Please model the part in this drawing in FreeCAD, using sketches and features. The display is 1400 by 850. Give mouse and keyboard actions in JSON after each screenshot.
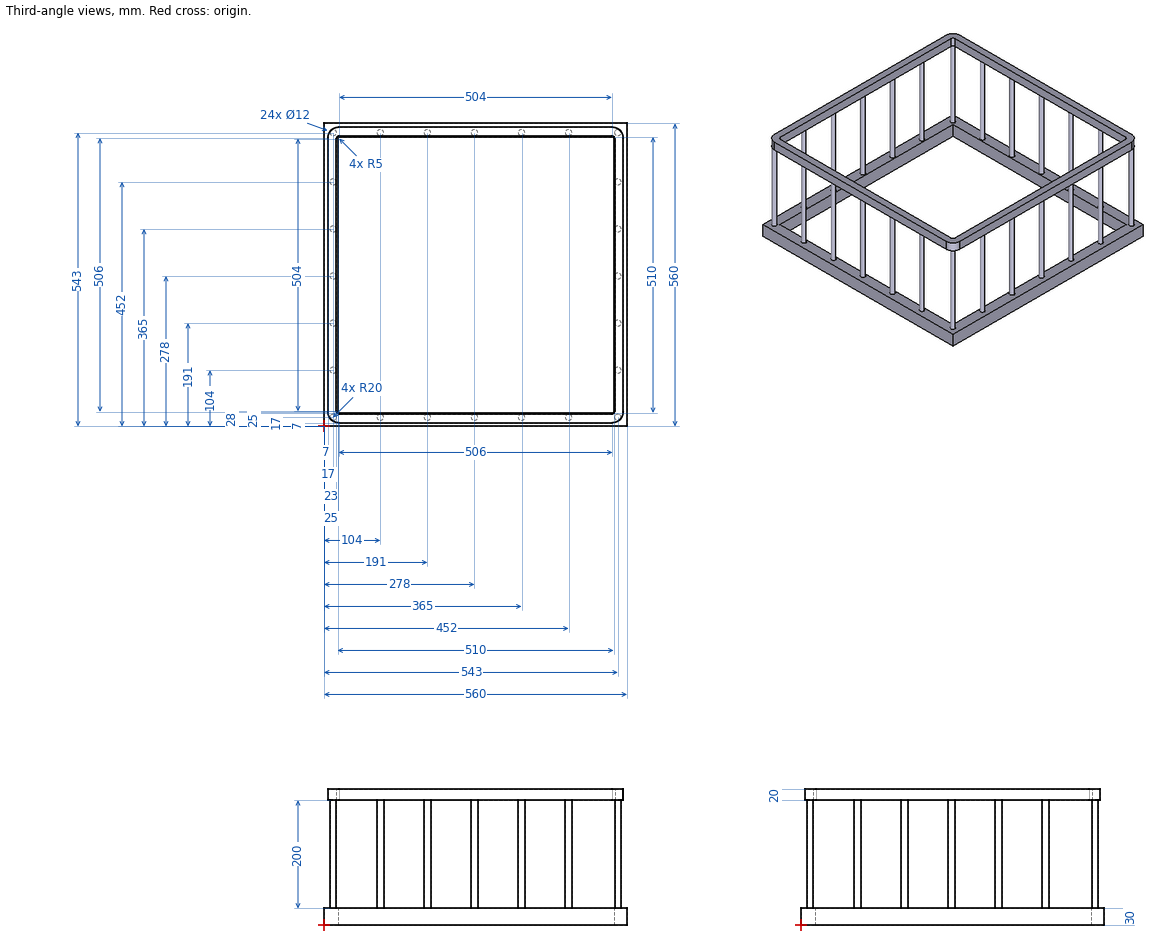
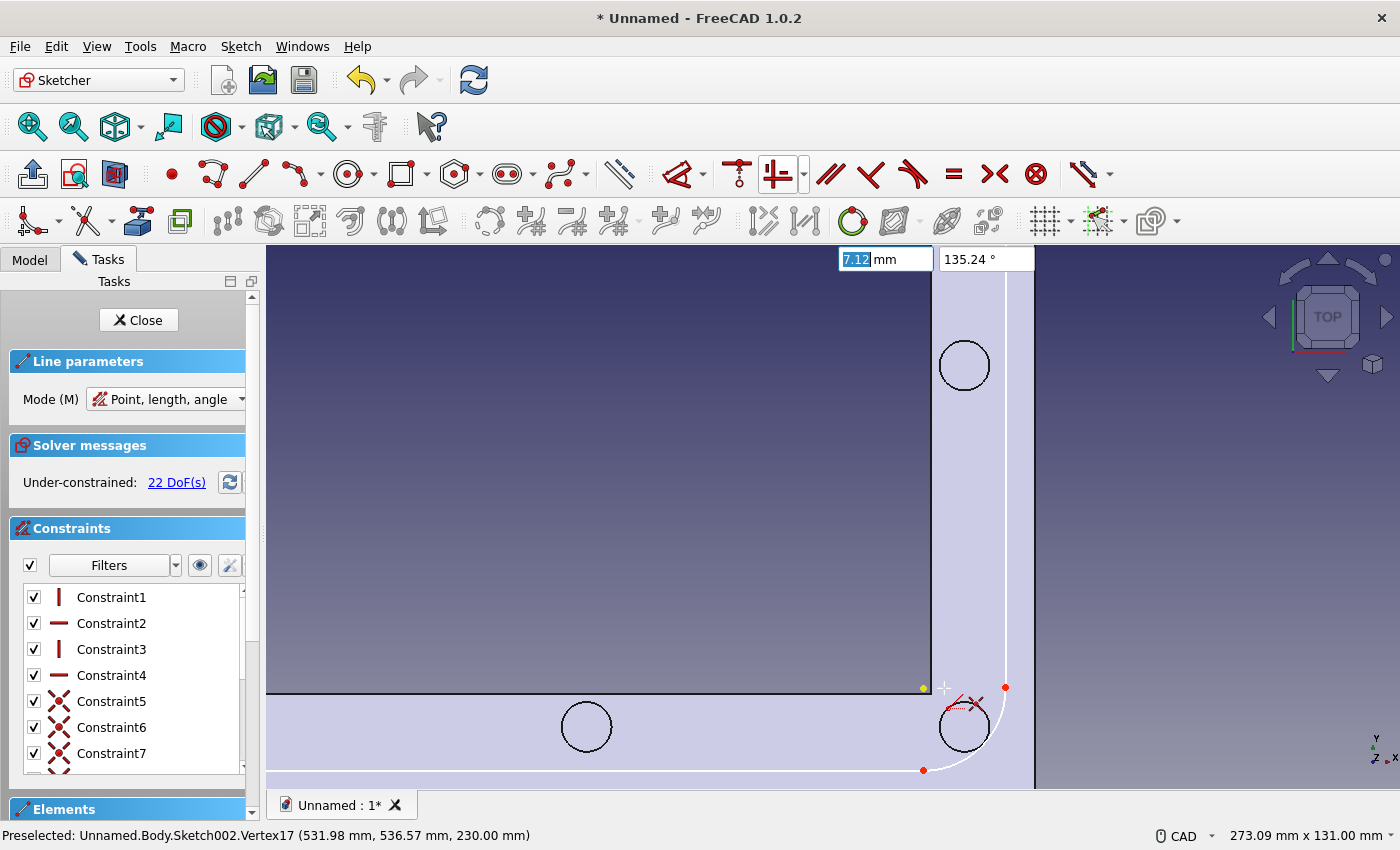
{"action": "left_click", "coordinate": [940, 681]}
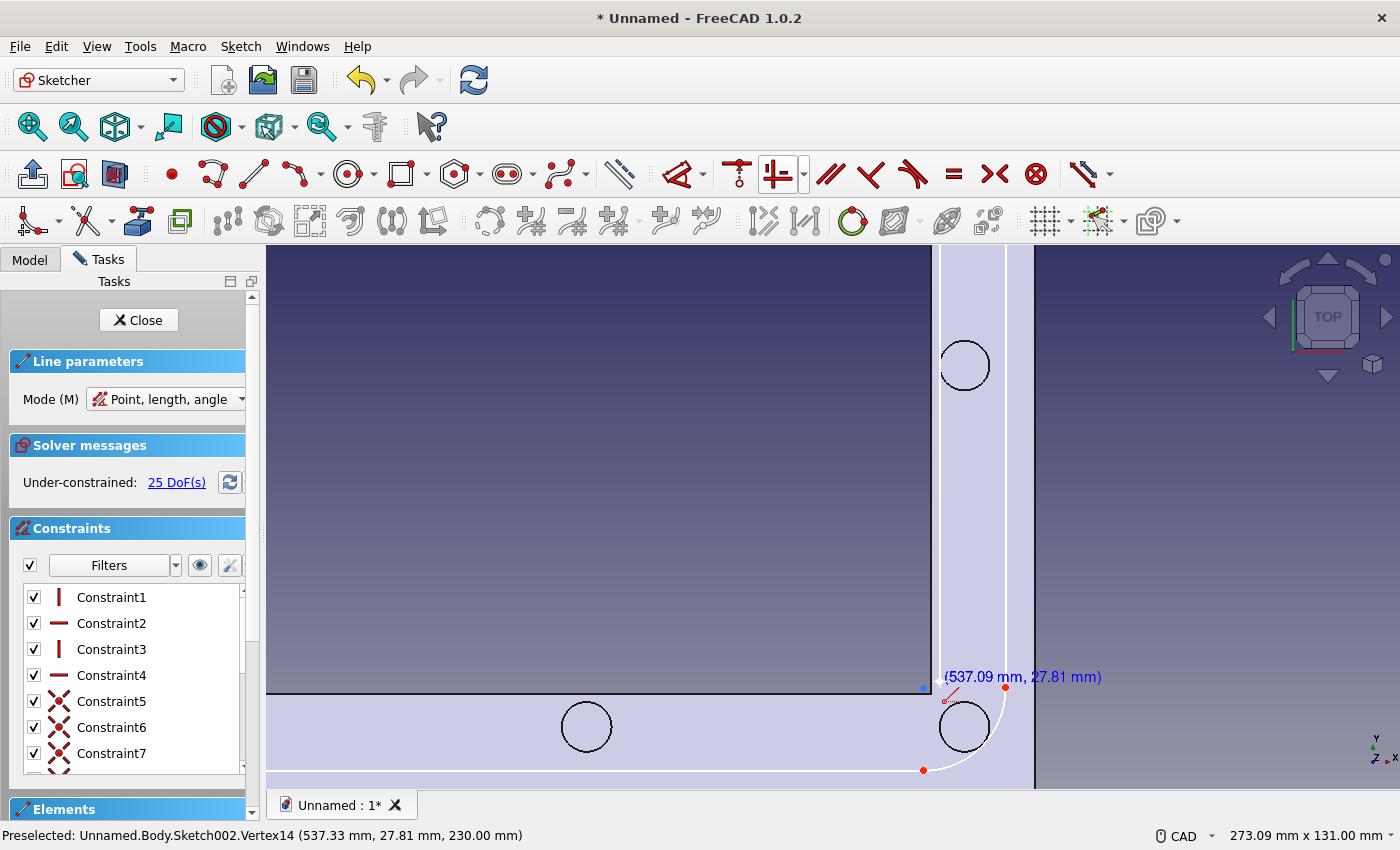
{"action": "left_click", "coordinate": [919, 702]}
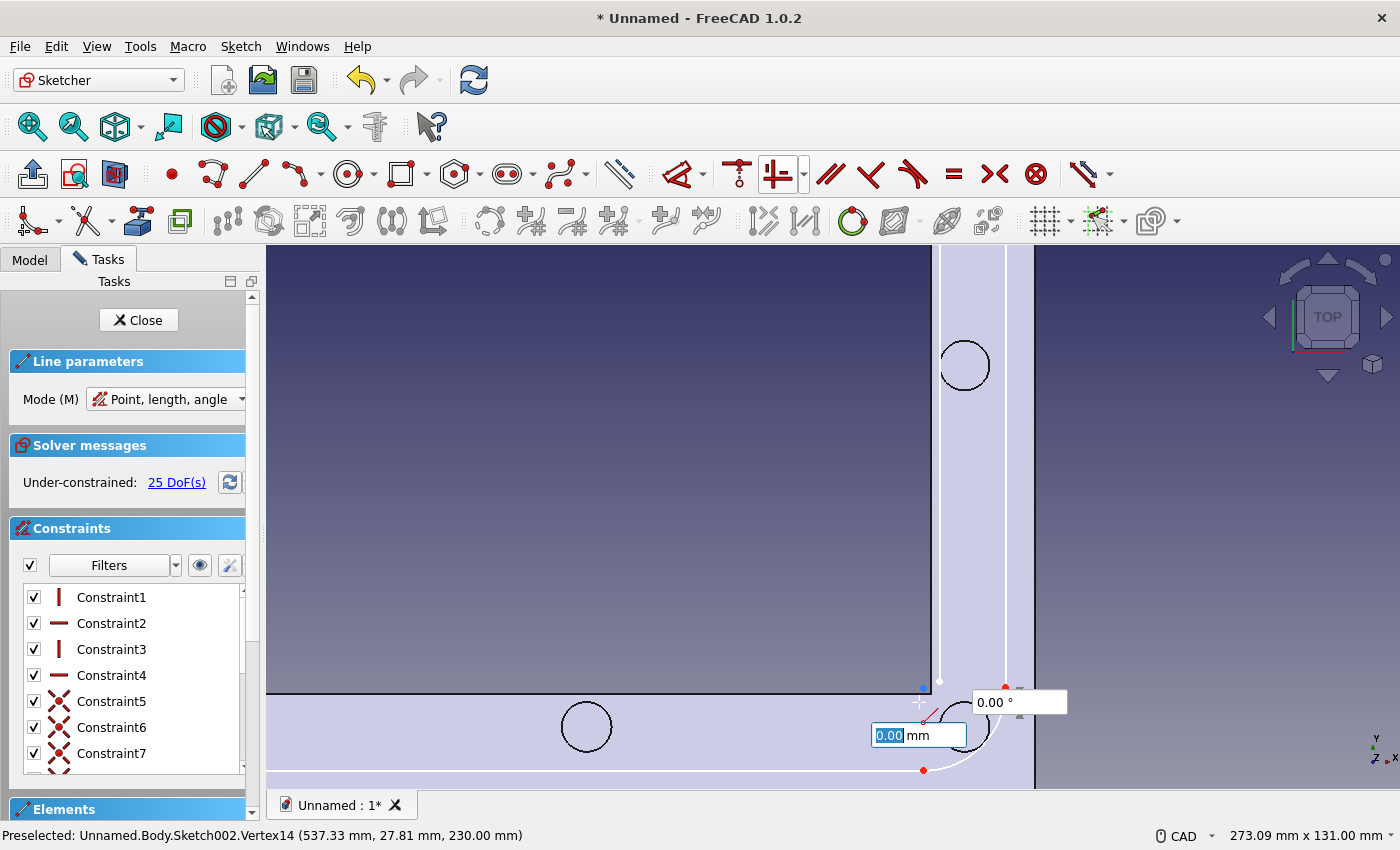
{"action": "scroll", "coordinate": [944, 689], "scroll_direction": "down", "scroll_amount": 9}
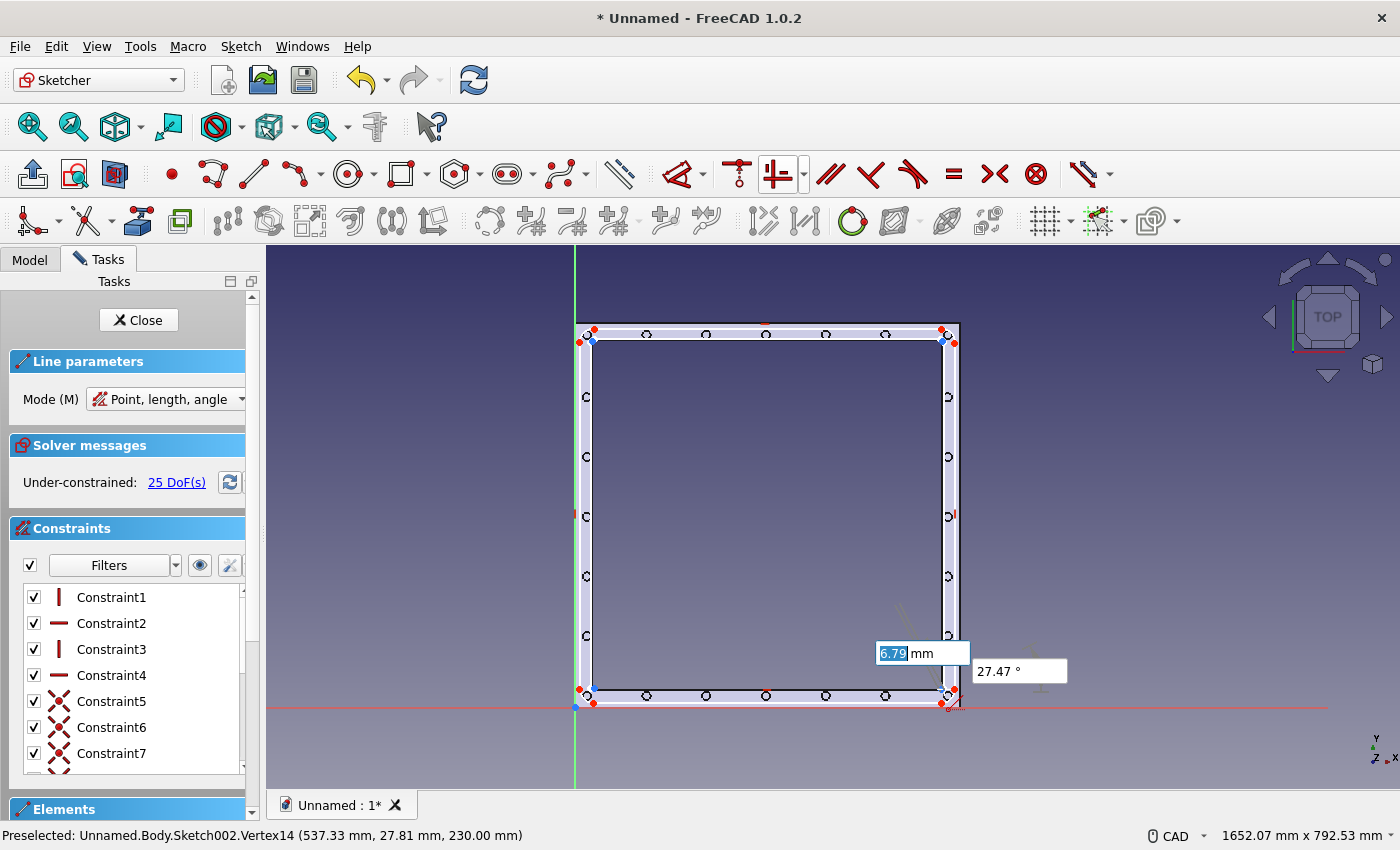
{"action": "scroll", "coordinate": [594, 692], "scroll_direction": "up", "scroll_amount": 9}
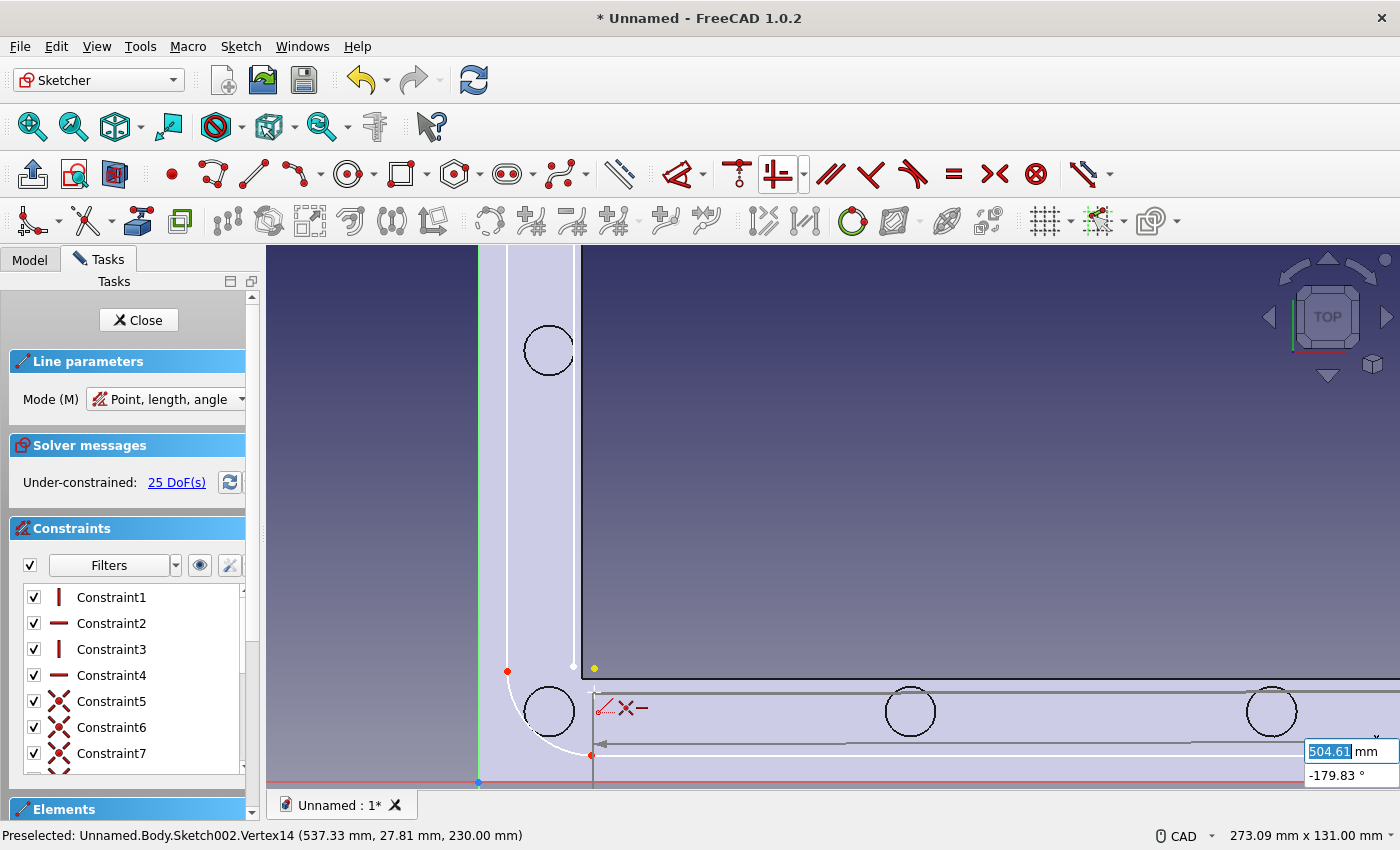
{"action": "left_click", "coordinate": [595, 687]}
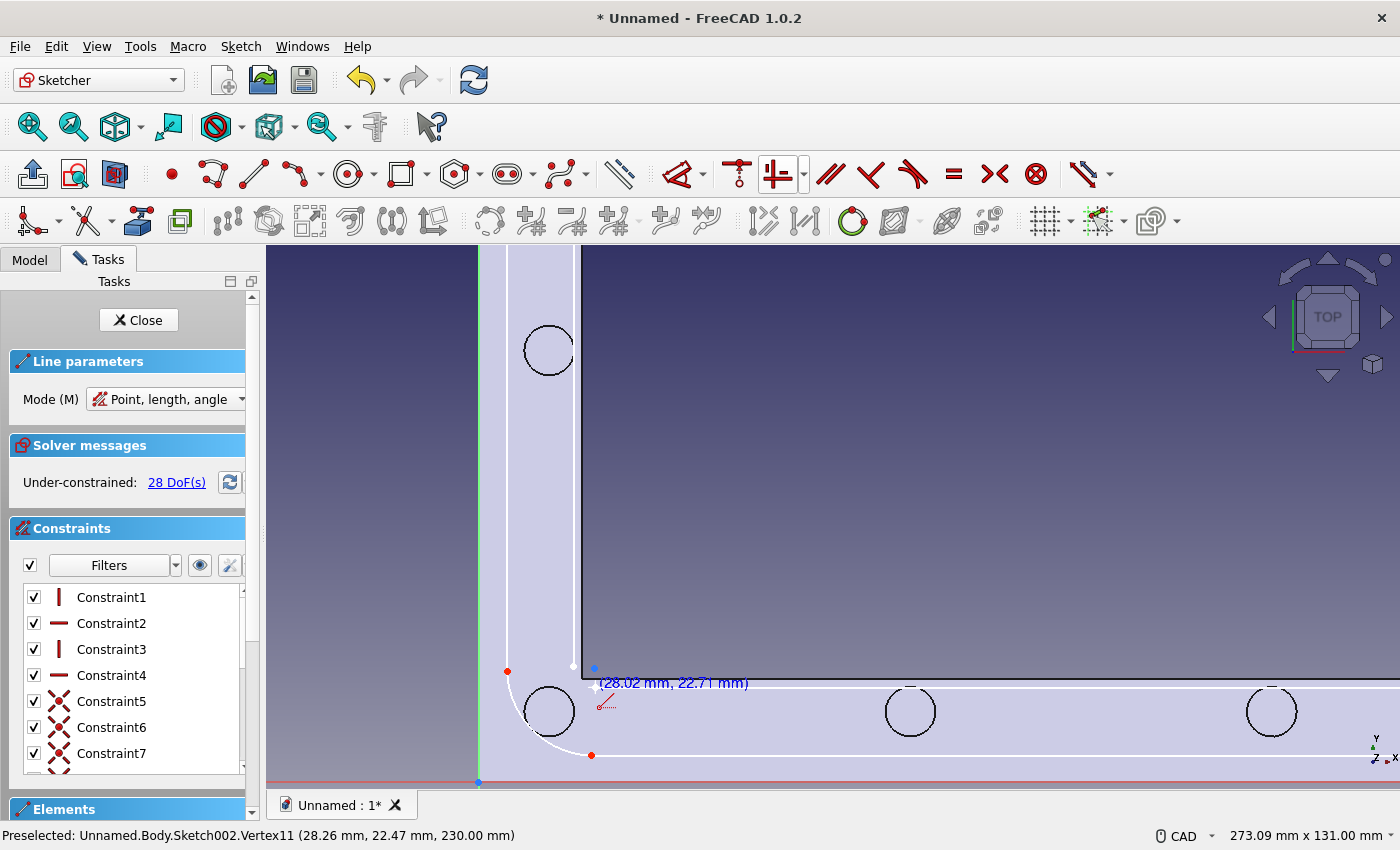
{"action": "left_click", "coordinate": [294, 174]}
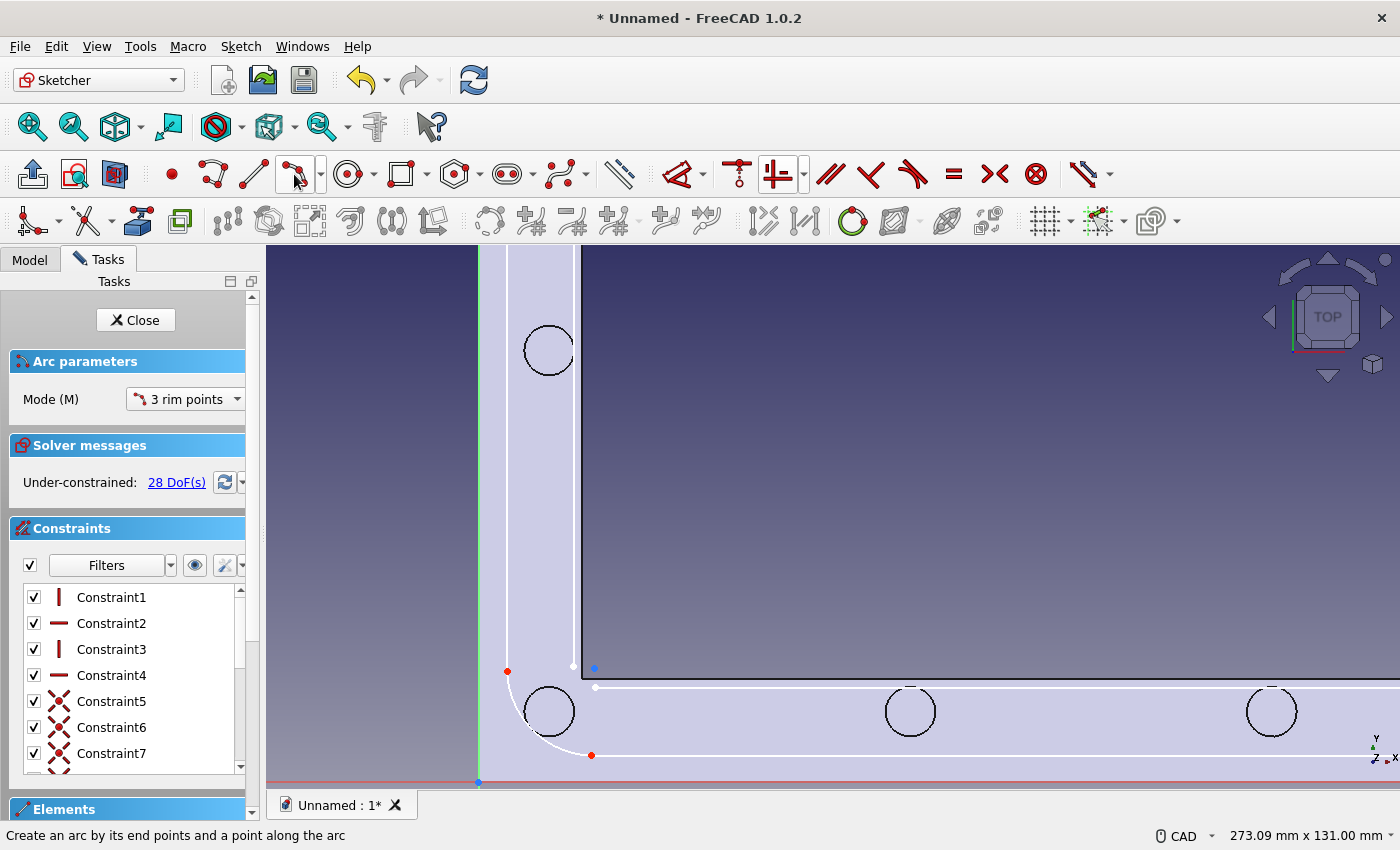
{"action": "scroll", "coordinate": [594, 692], "scroll_direction": "down", "scroll_amount": 9}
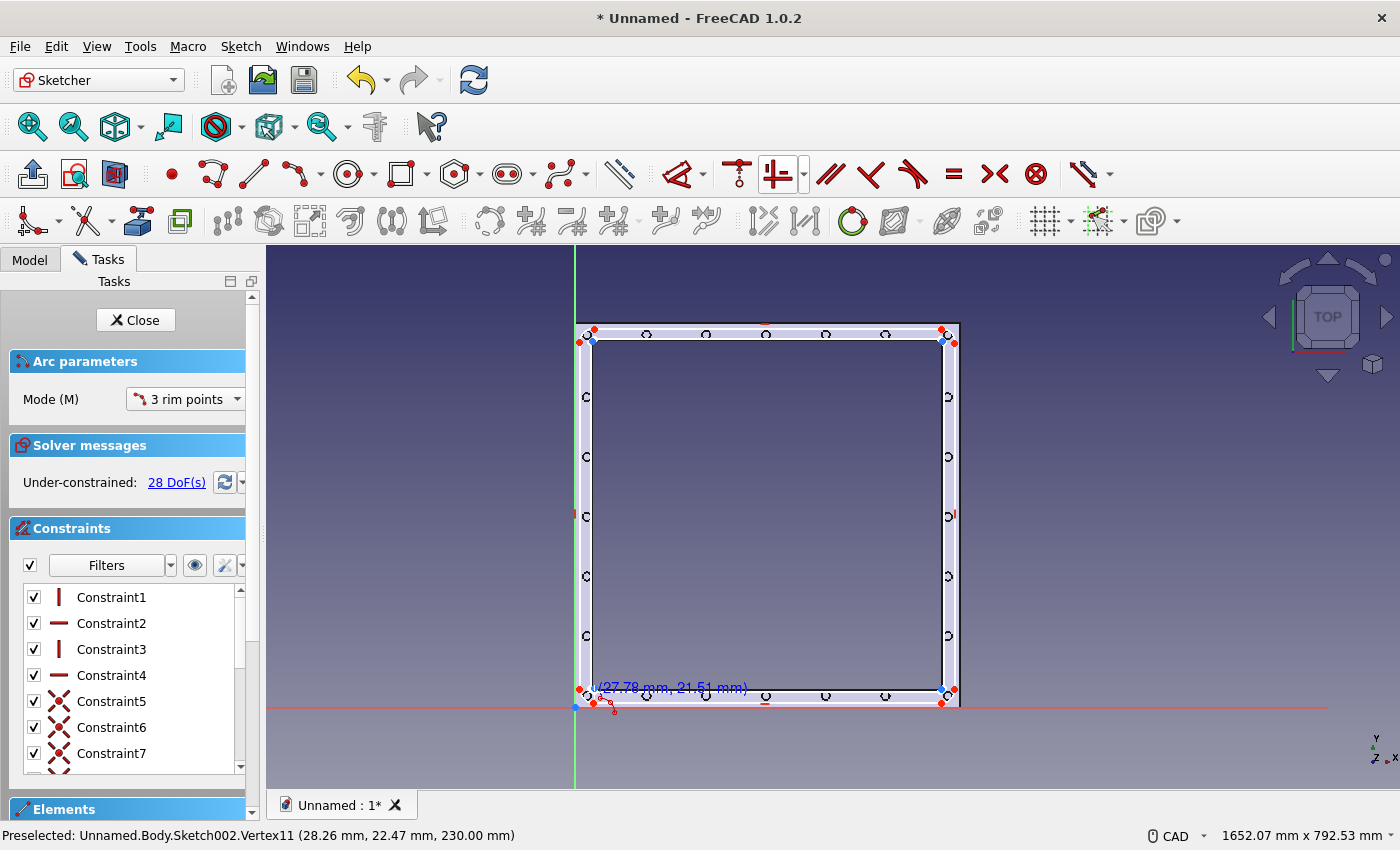
{"action": "scroll", "coordinate": [591, 342], "scroll_direction": "up", "scroll_amount": 9}